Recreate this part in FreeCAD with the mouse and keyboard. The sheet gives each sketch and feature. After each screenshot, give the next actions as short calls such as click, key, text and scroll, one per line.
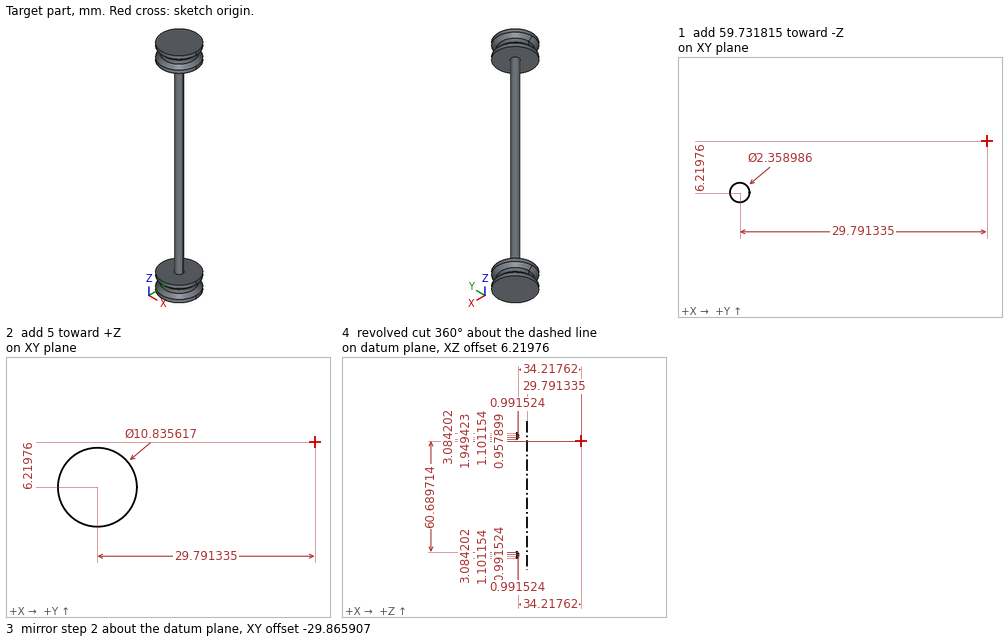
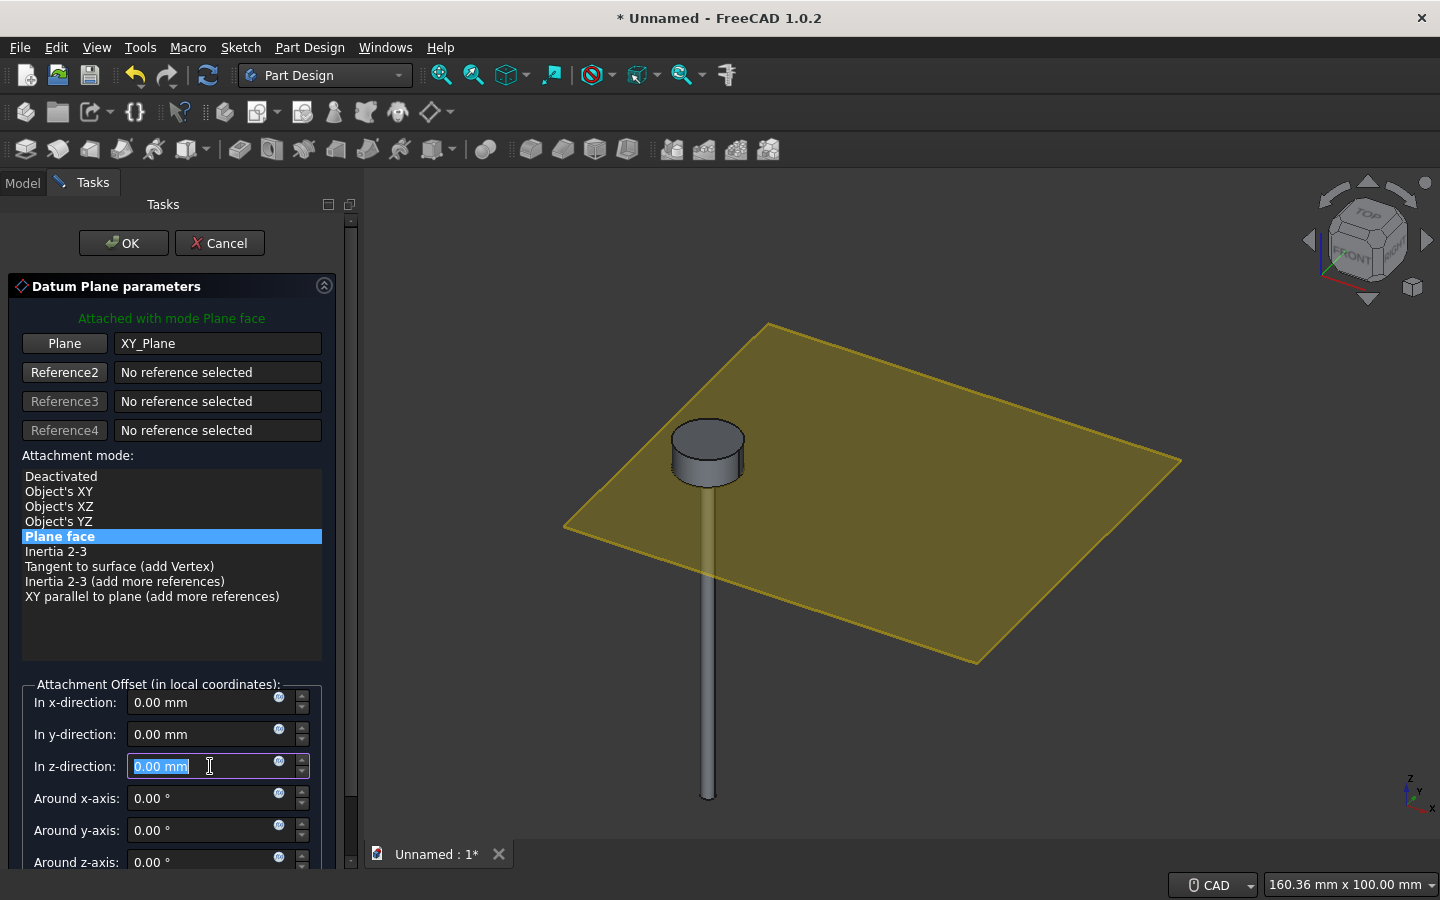
text(-29.865907)
key(Tab)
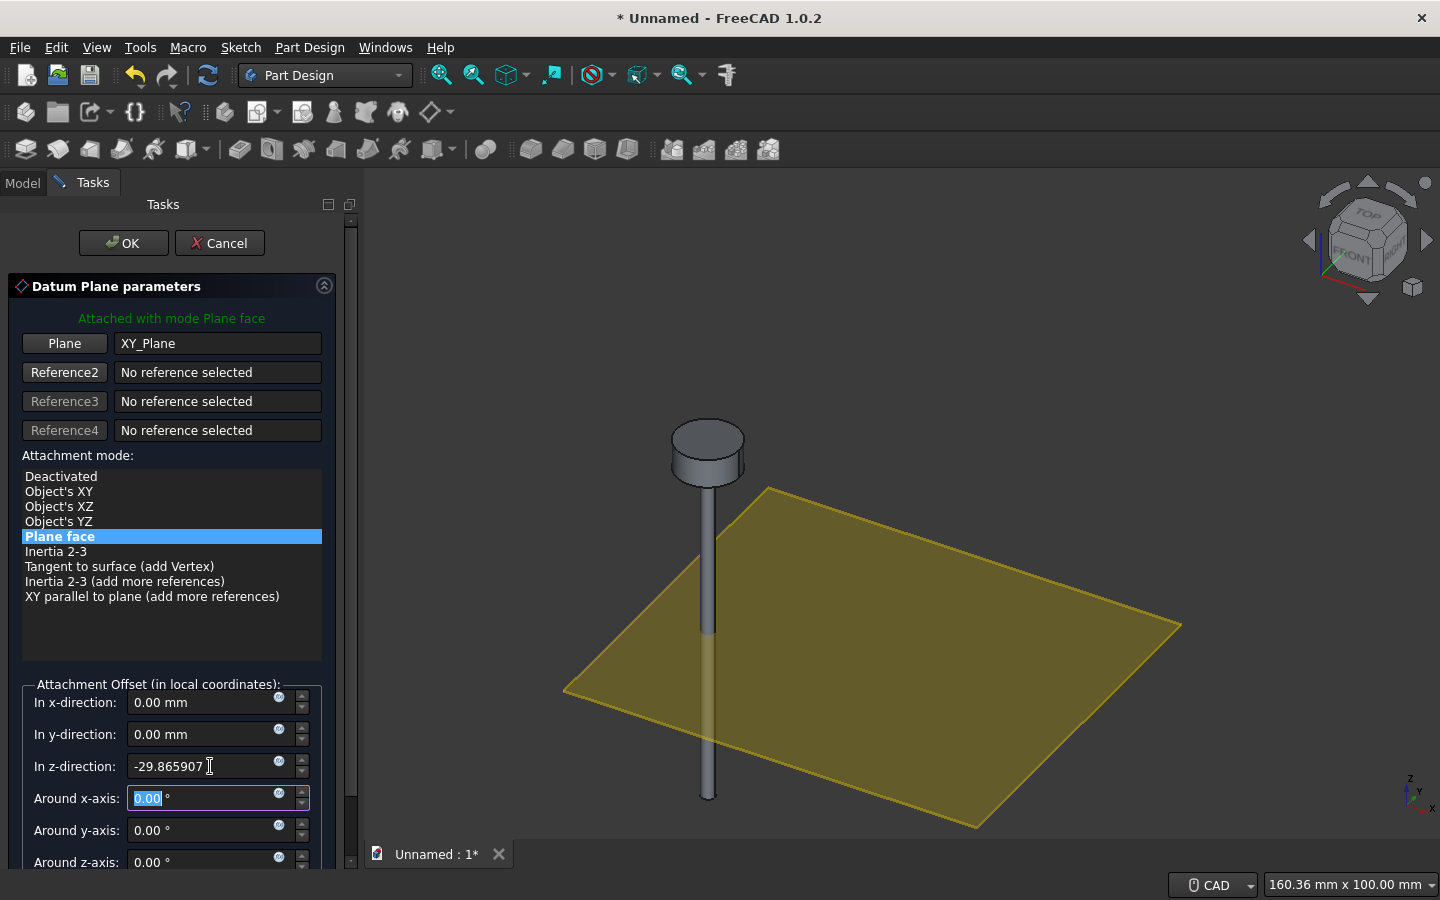
click(124, 243)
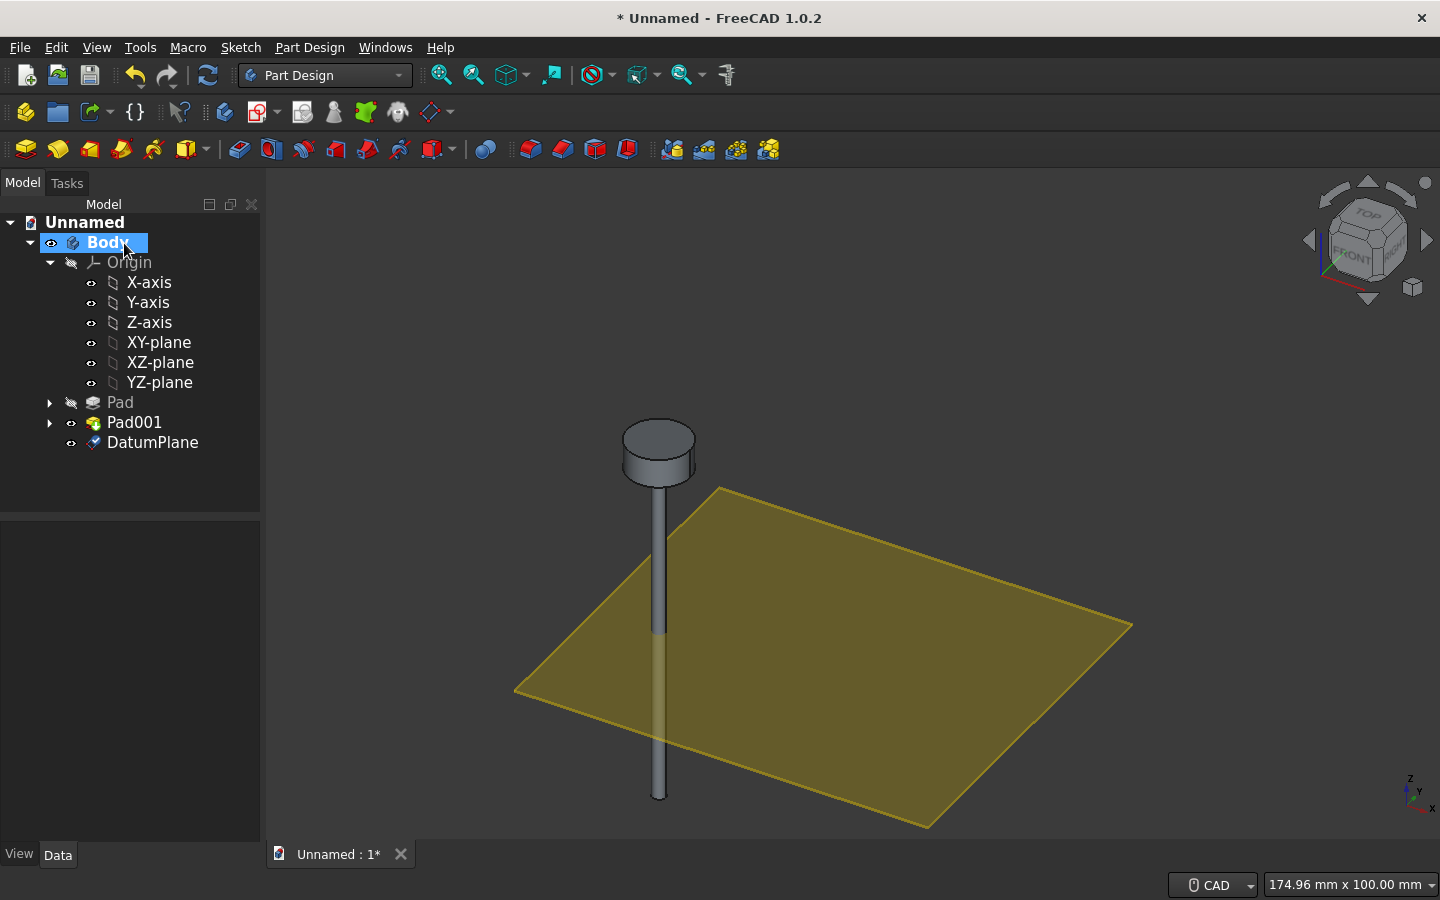
click(116, 423)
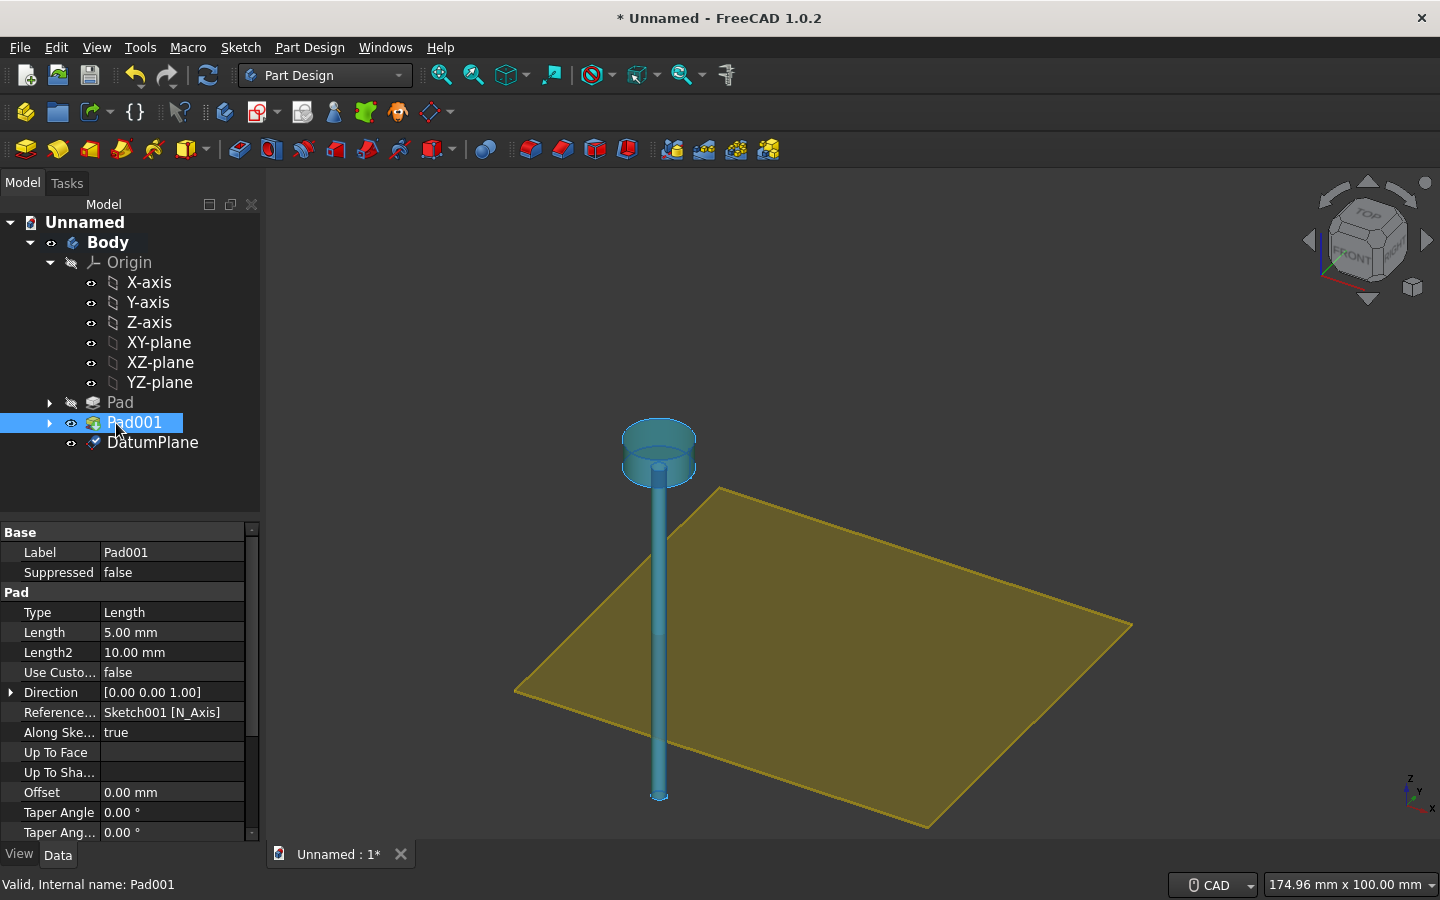
click(672, 150)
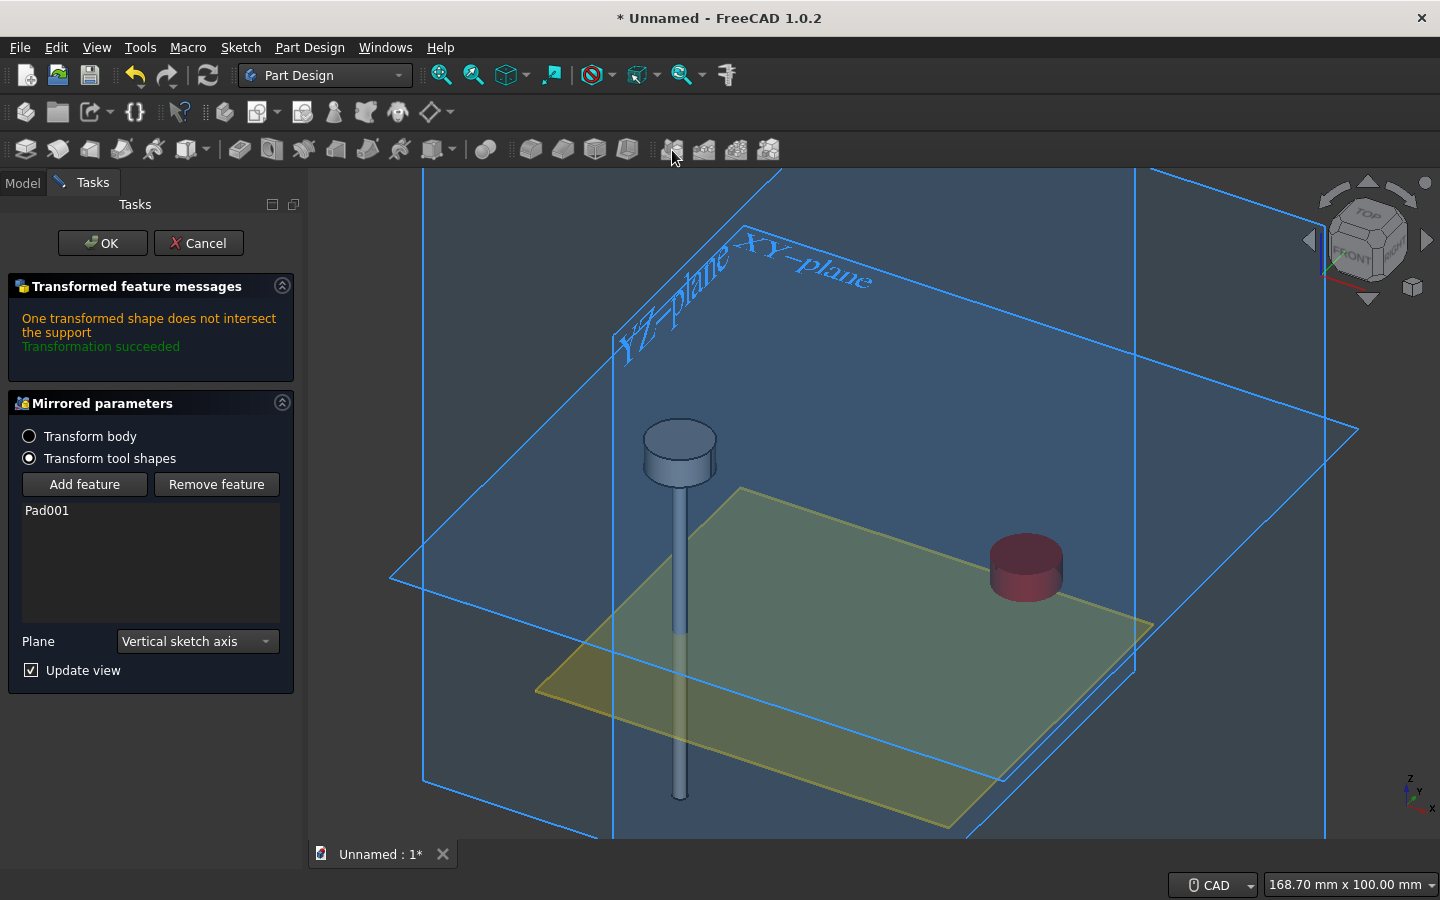
click(198, 642)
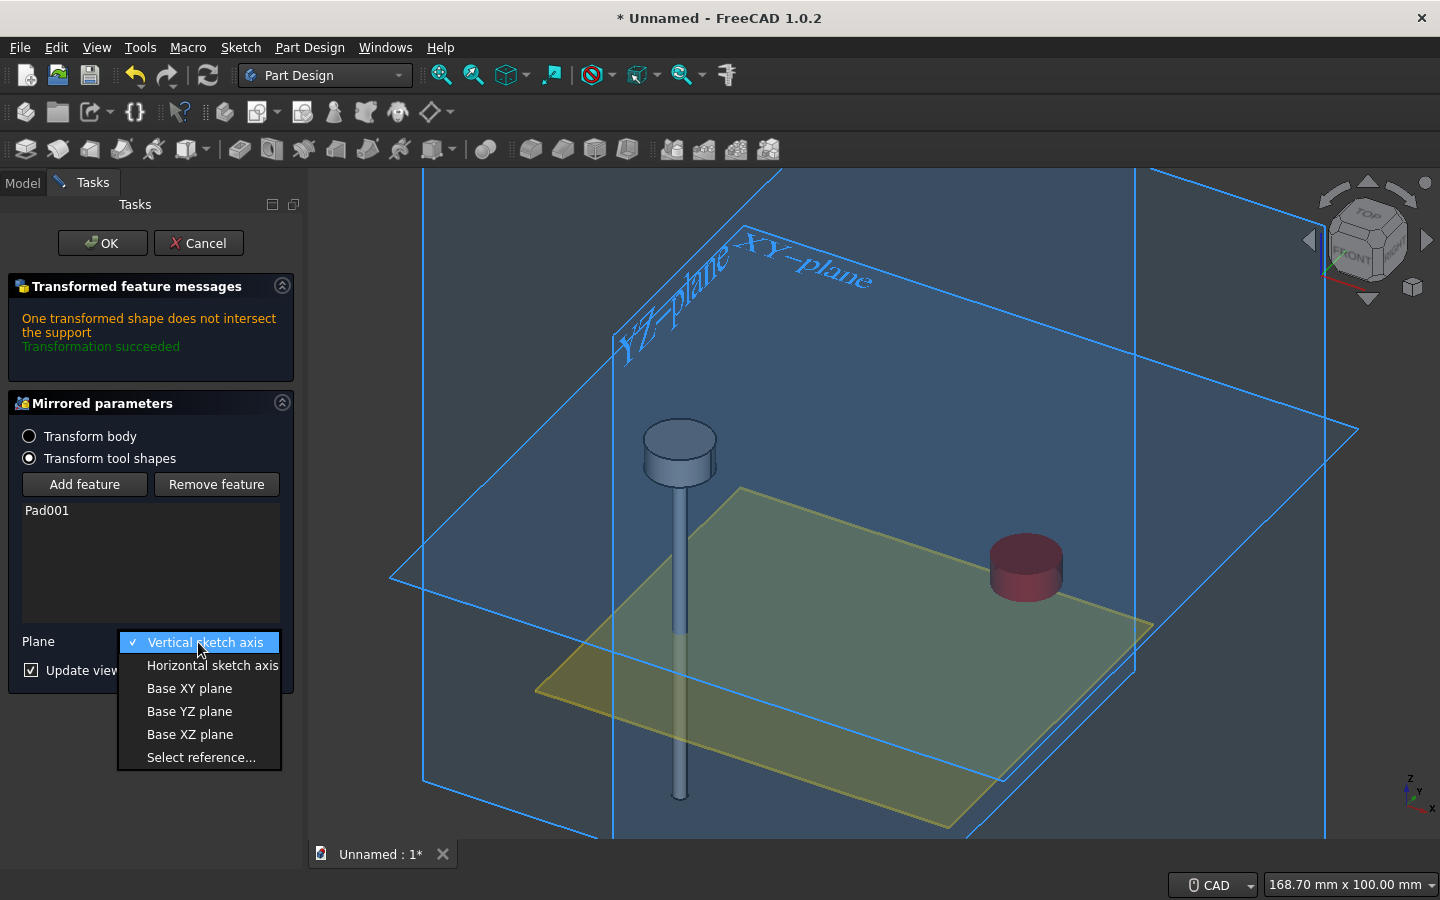
click(198, 758)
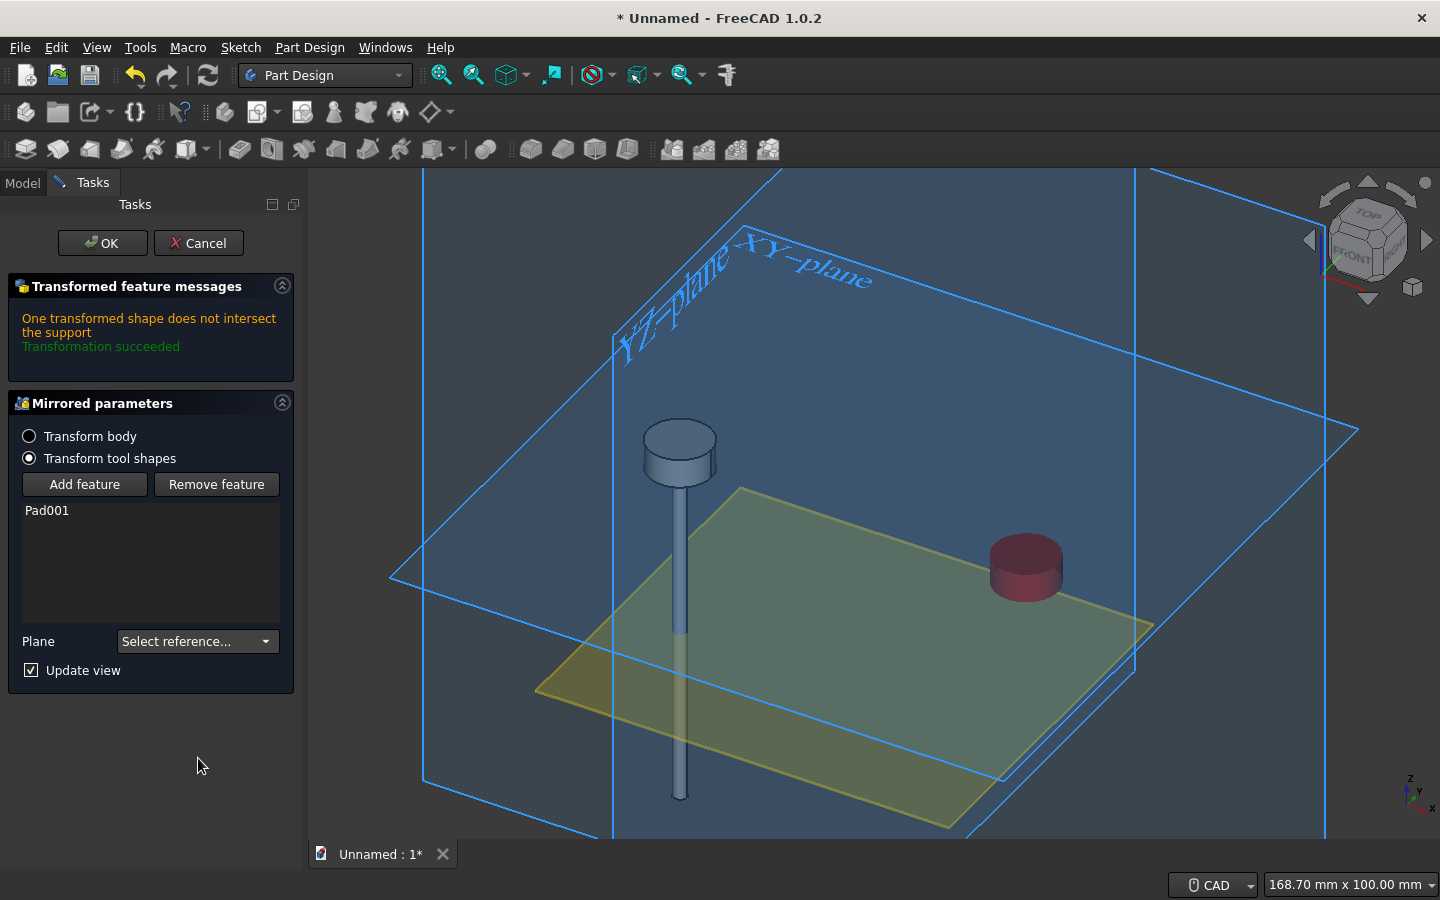
click(23, 182)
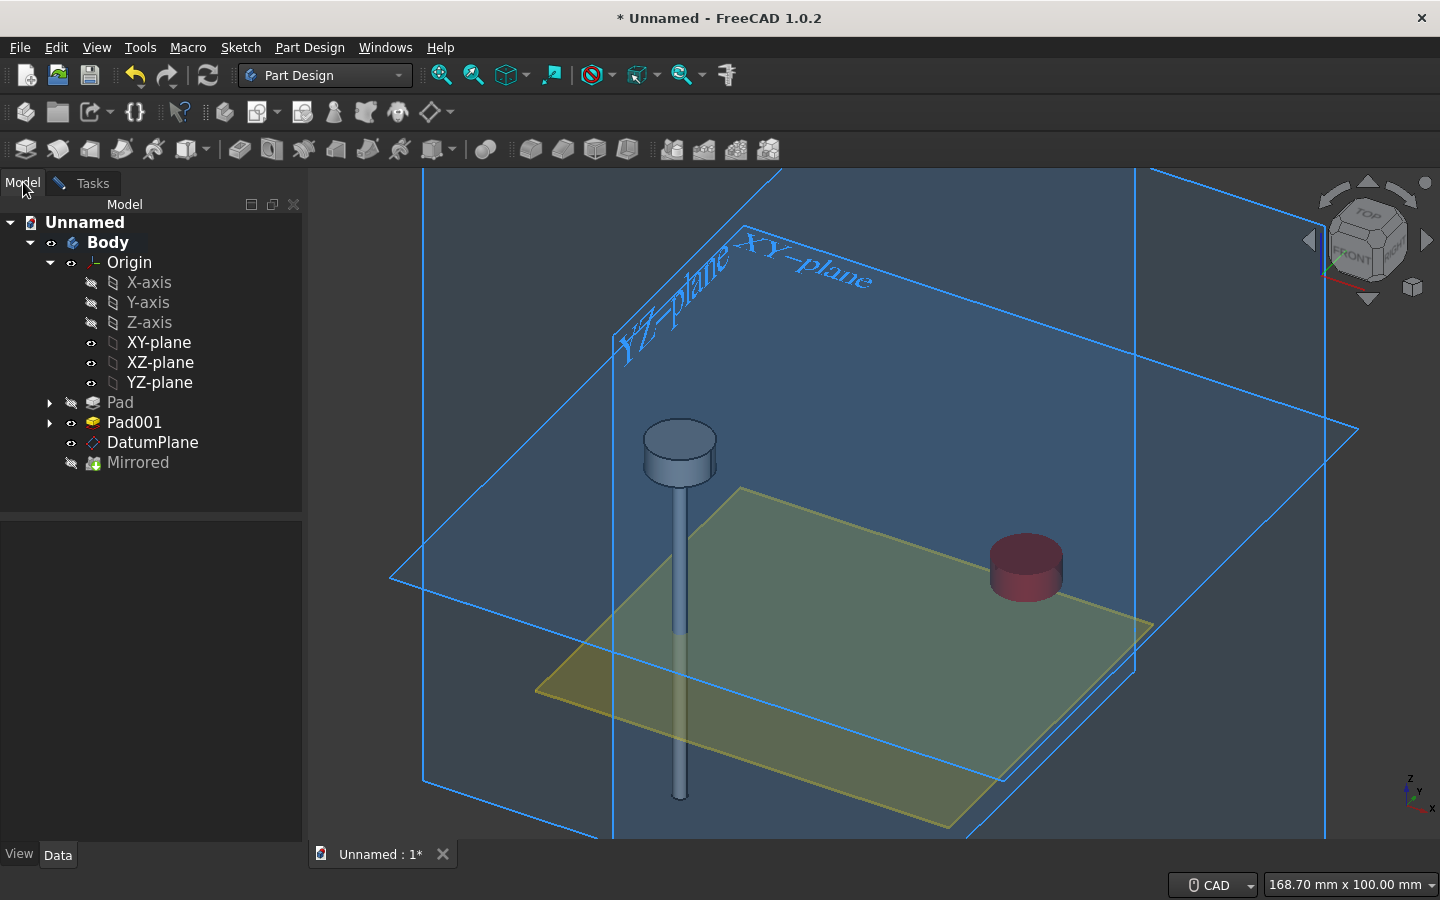
click(116, 443)